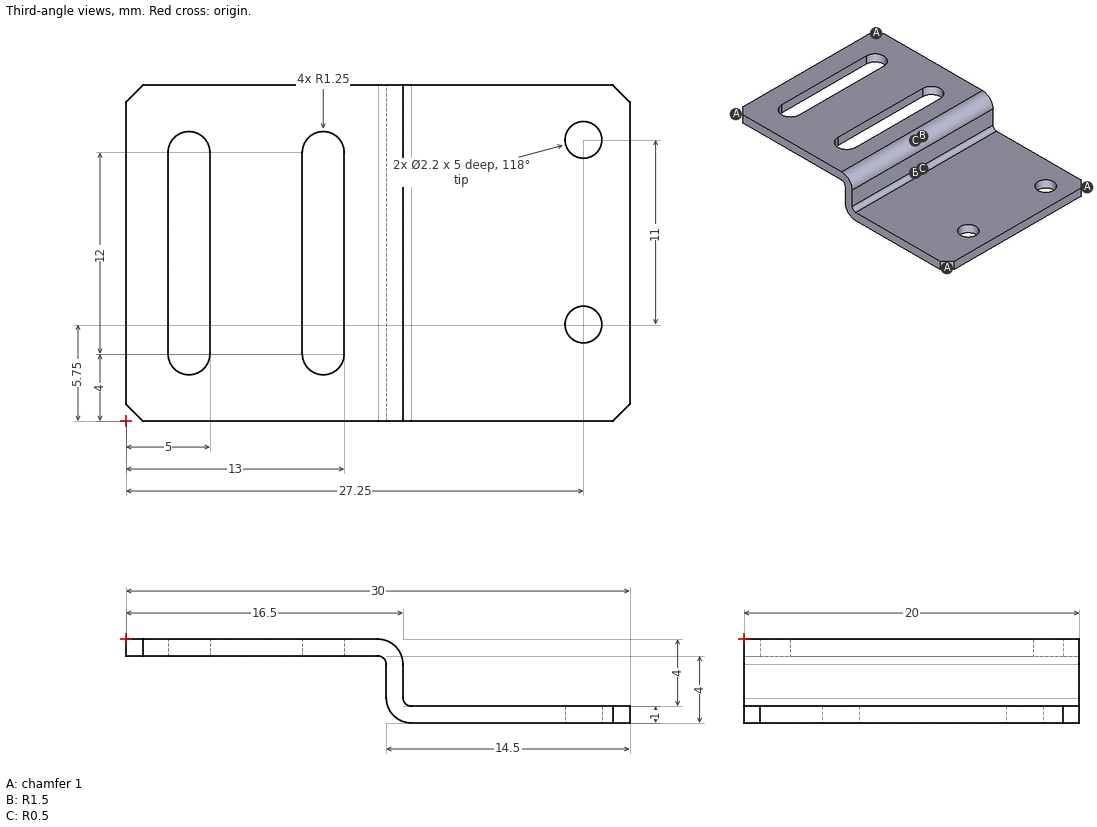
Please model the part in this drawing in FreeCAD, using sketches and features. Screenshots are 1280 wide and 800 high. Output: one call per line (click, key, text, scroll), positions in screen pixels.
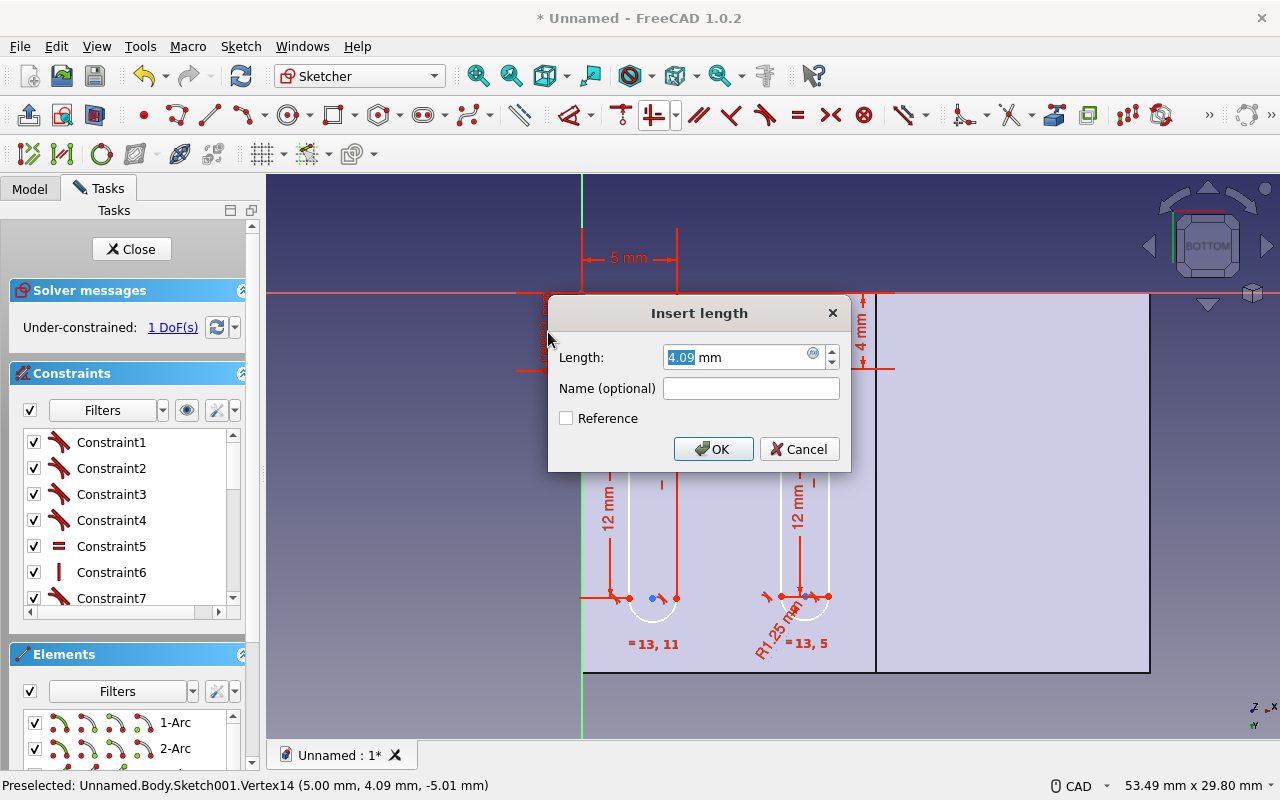
text(4)
key(Return)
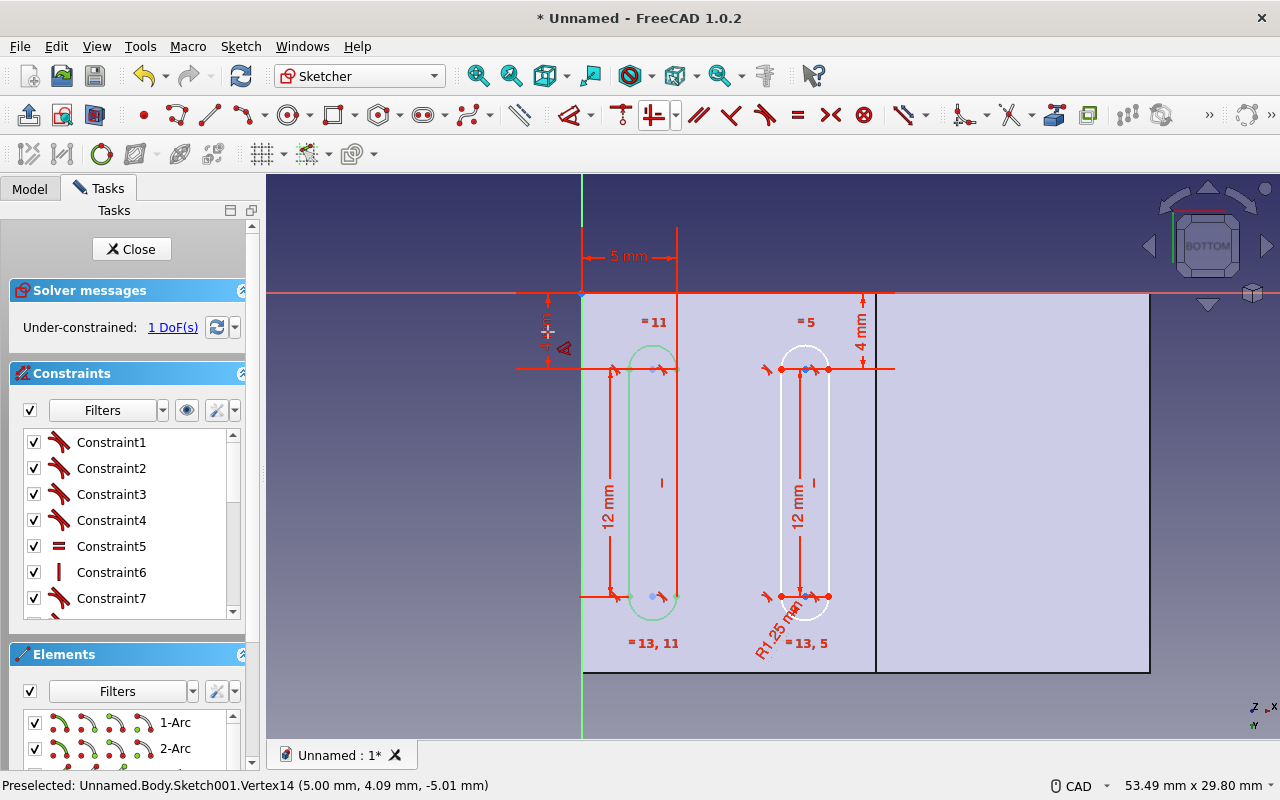
click(829, 597)
click(705, 259)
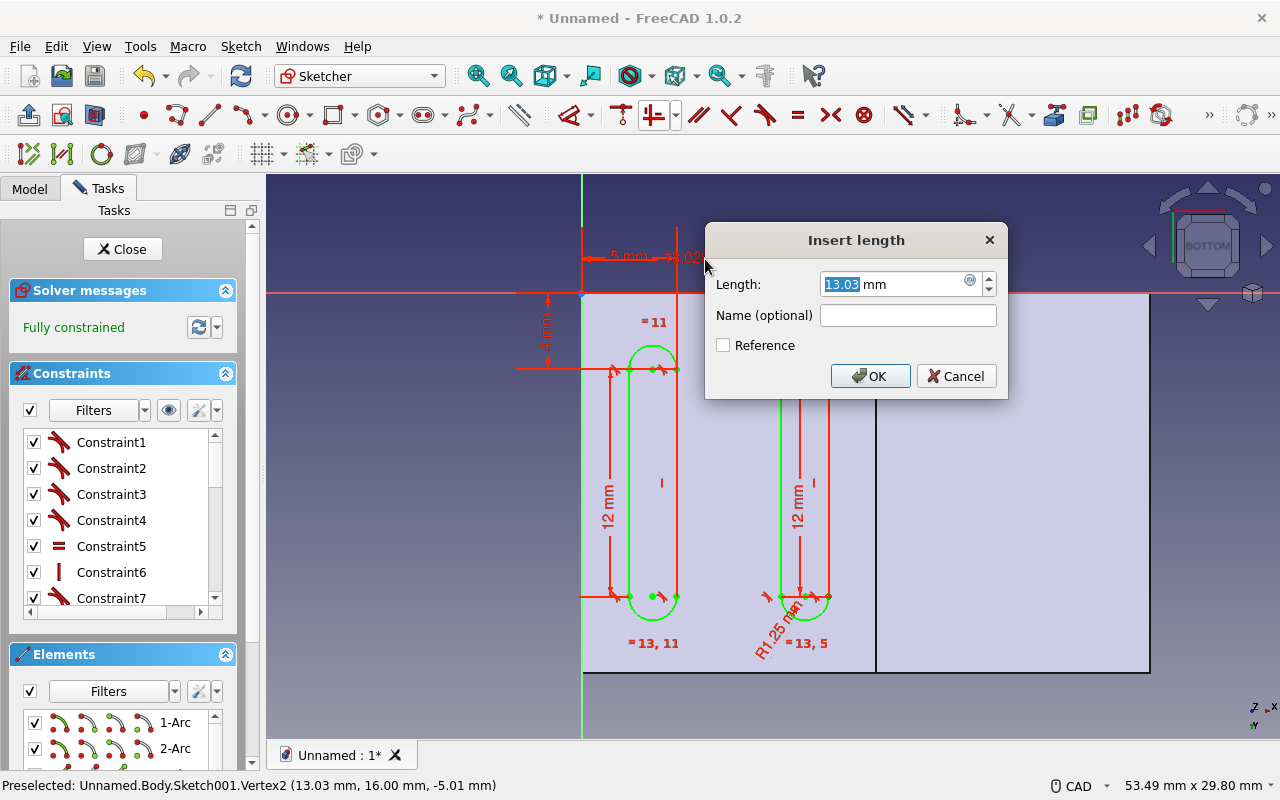
text(13)
key(Return)
key(Escape)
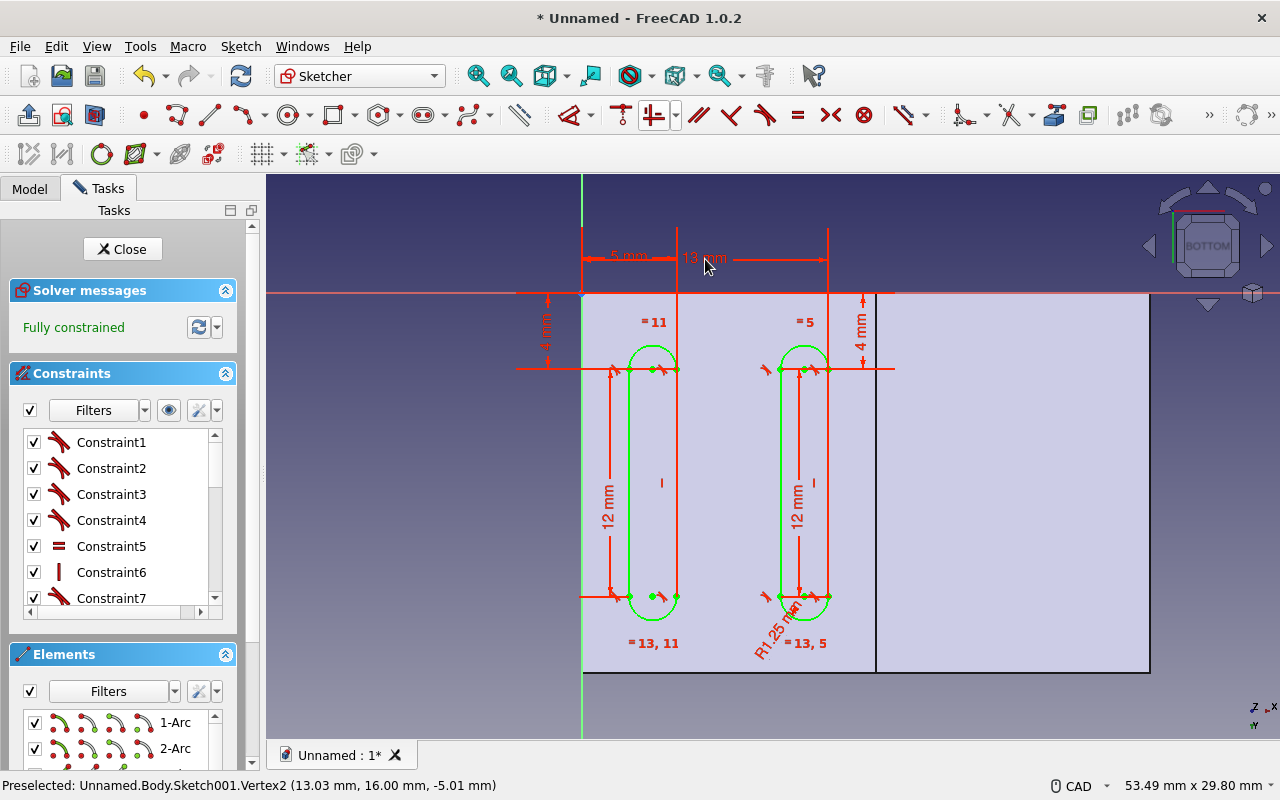
click(123, 249)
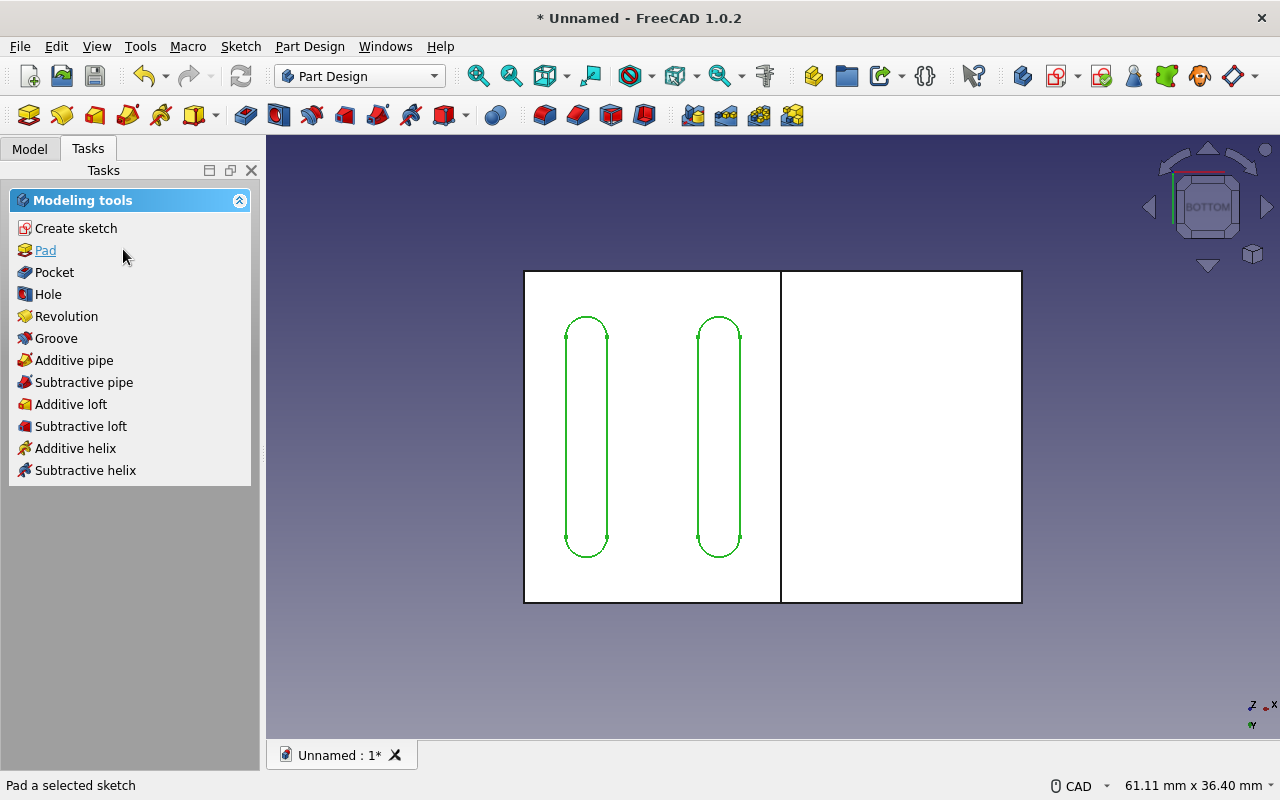
click(246, 116)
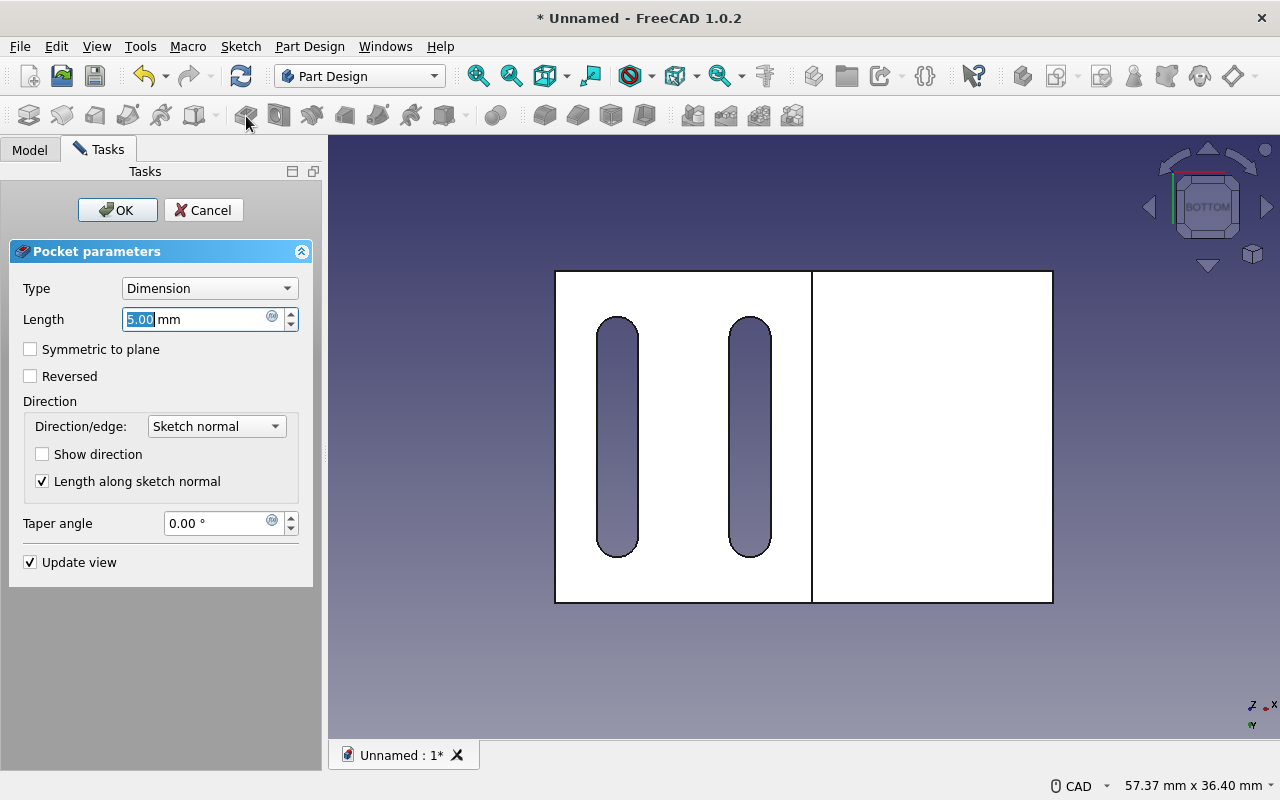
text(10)
key(Tab)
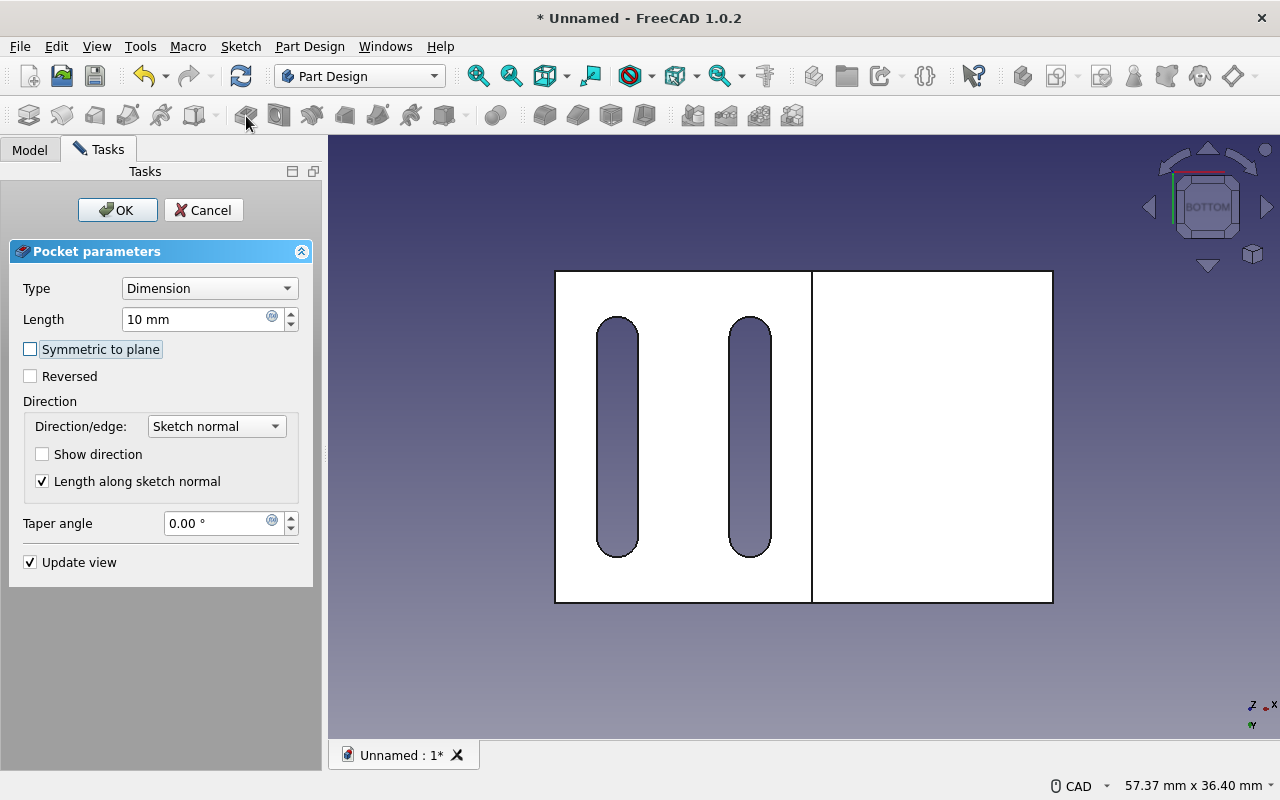
click(118, 210)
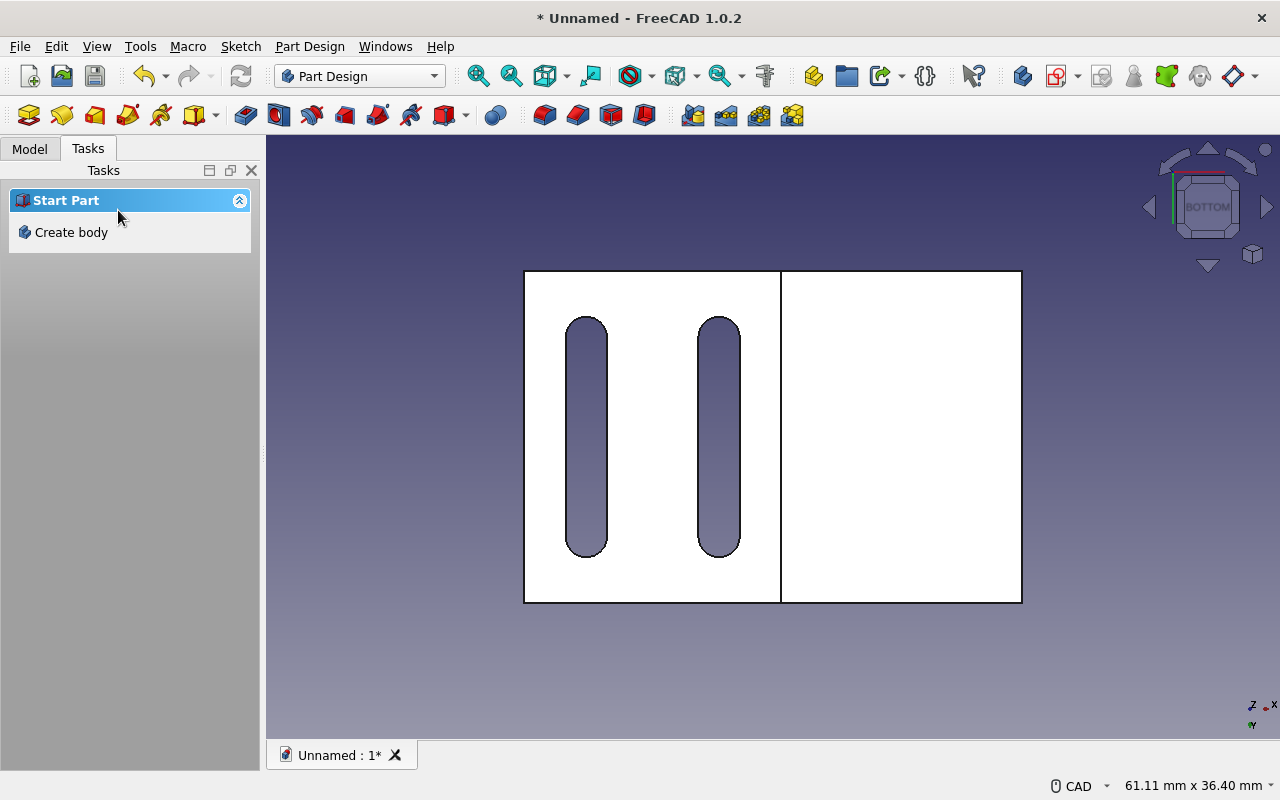
scroll(524, 270, up, 5)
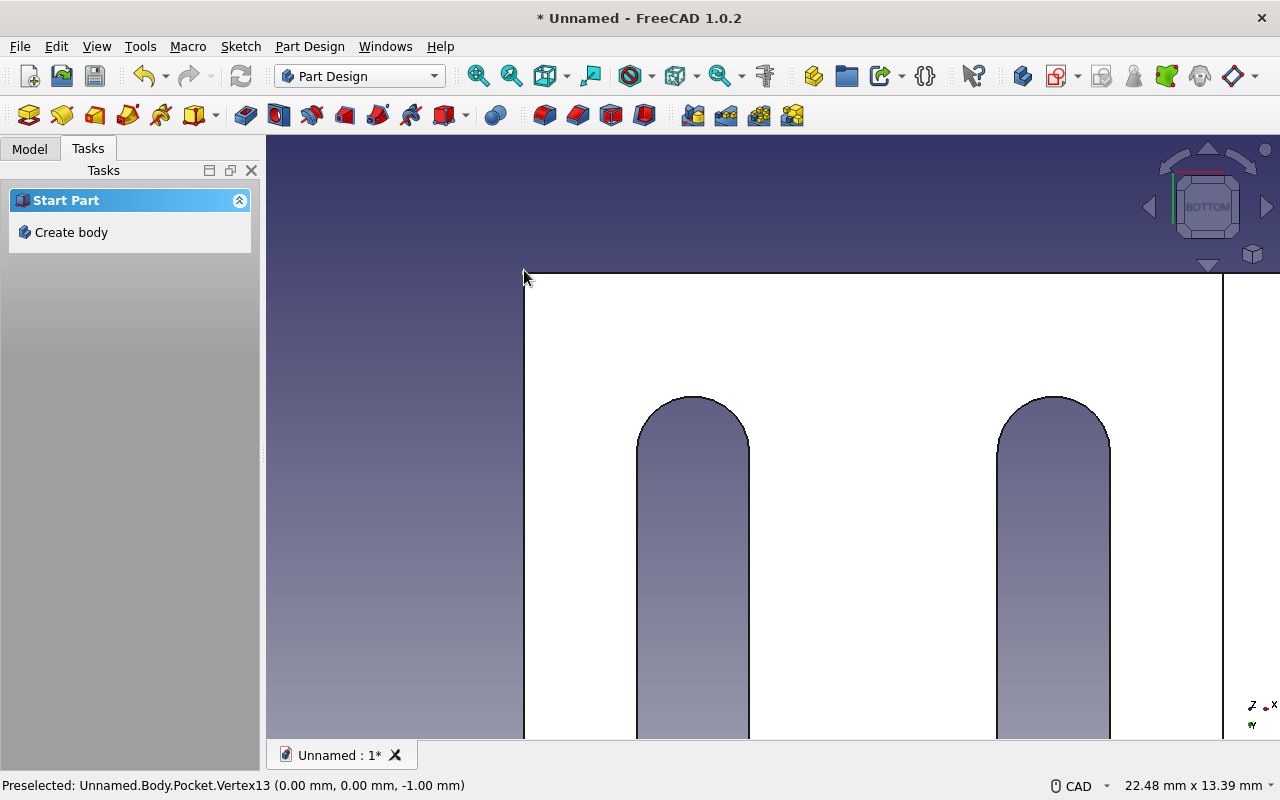
click(479, 76)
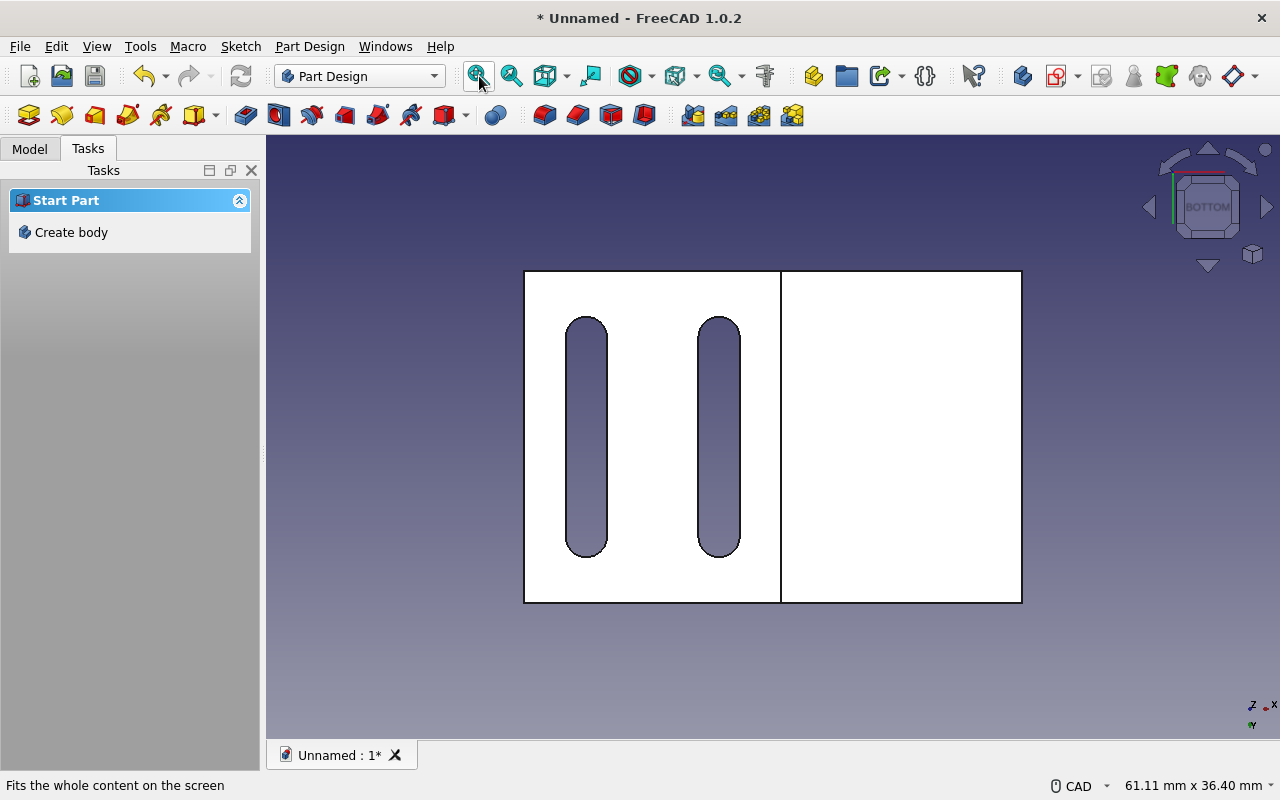
key(0)